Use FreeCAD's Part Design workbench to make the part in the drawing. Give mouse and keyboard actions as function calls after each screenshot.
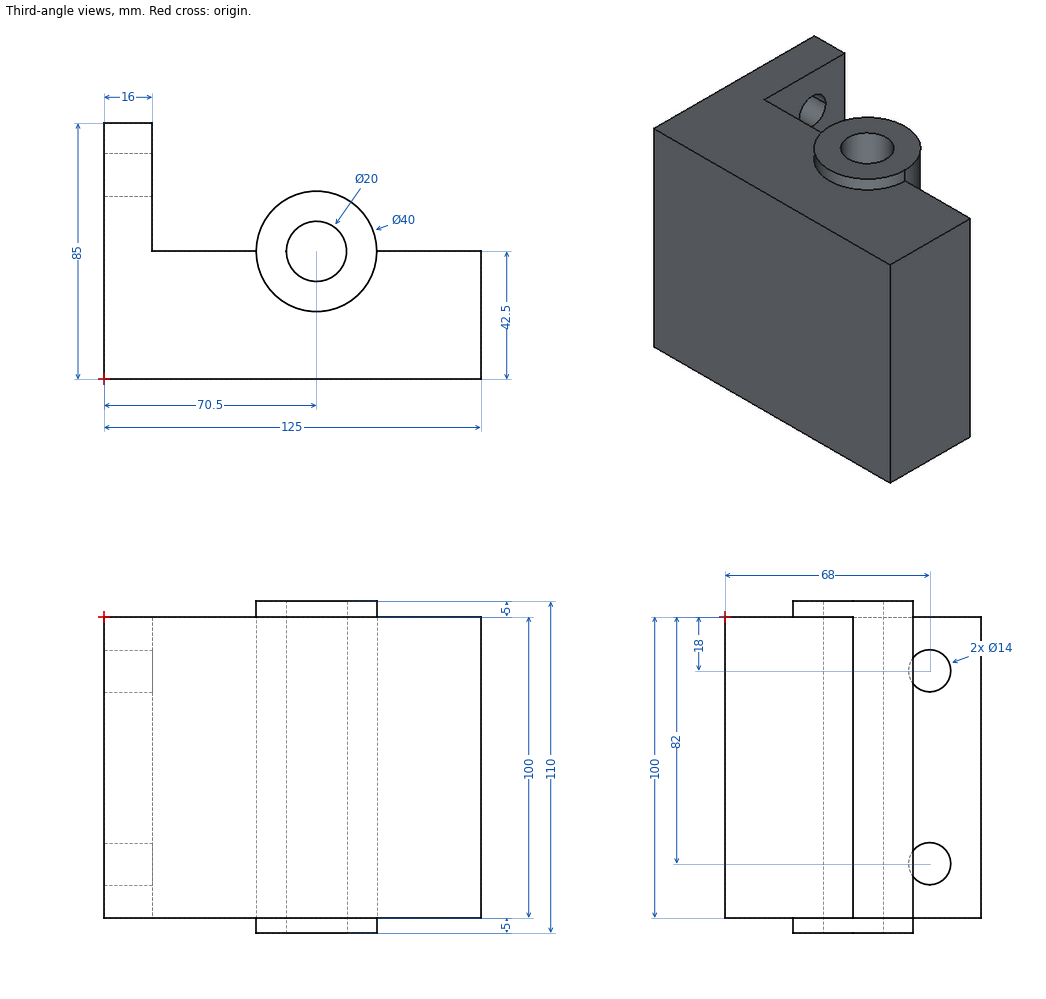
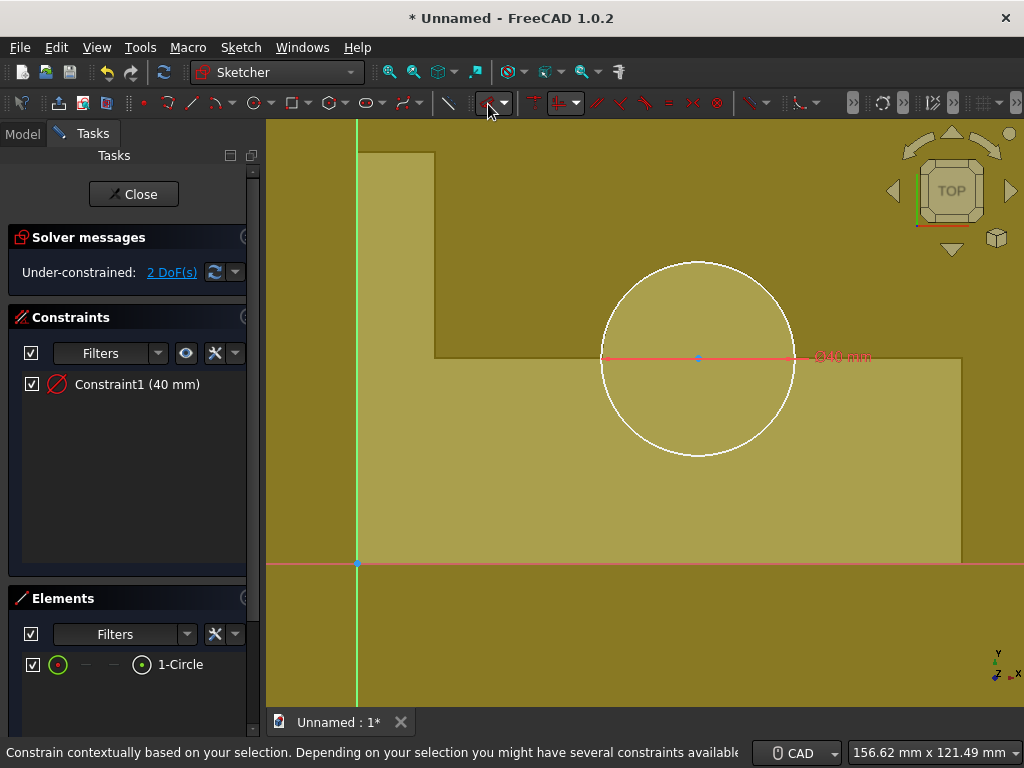
click(698, 359)
click(528, 598)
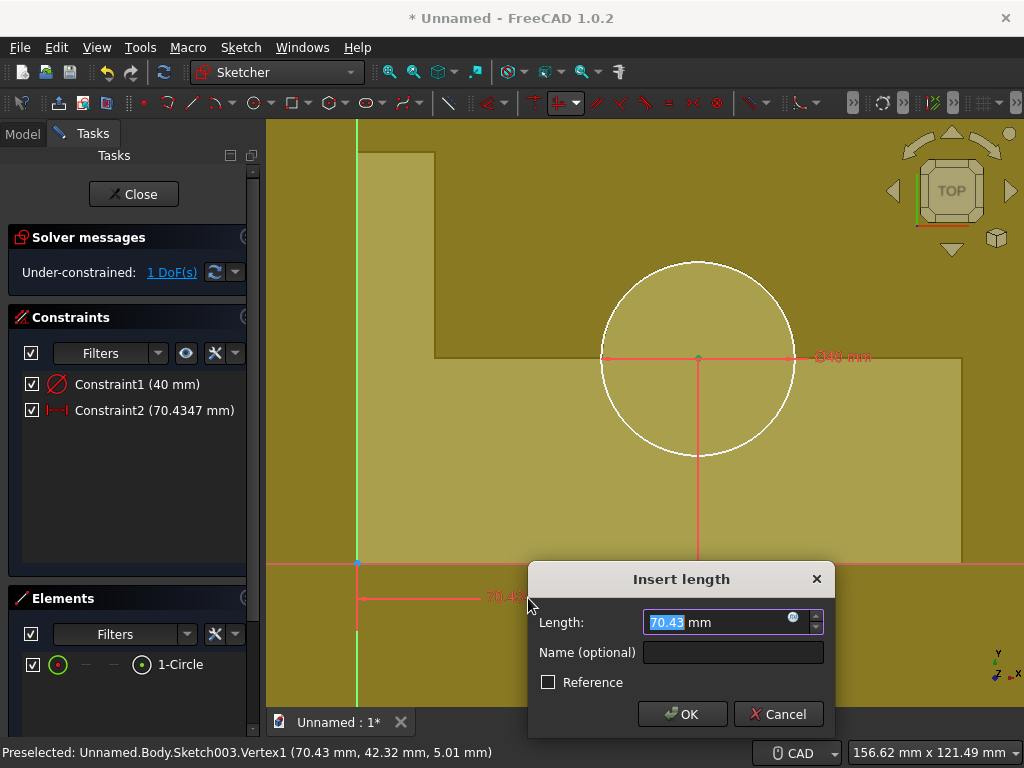
text(70.5)
key(Return)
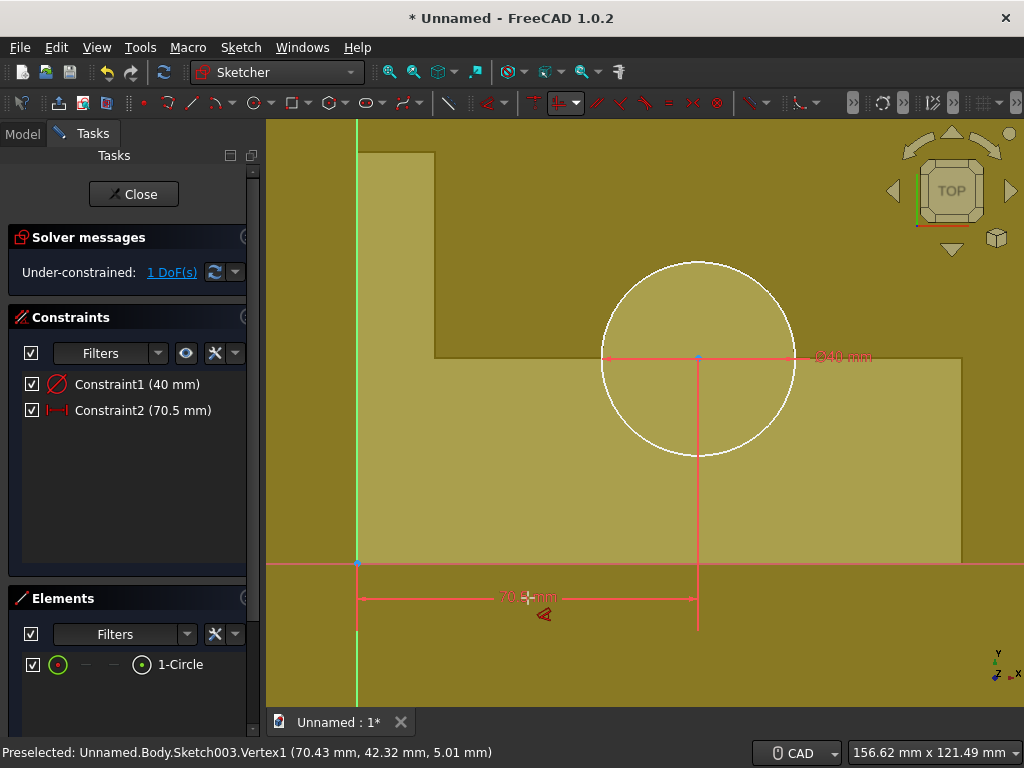
click(698, 359)
click(323, 461)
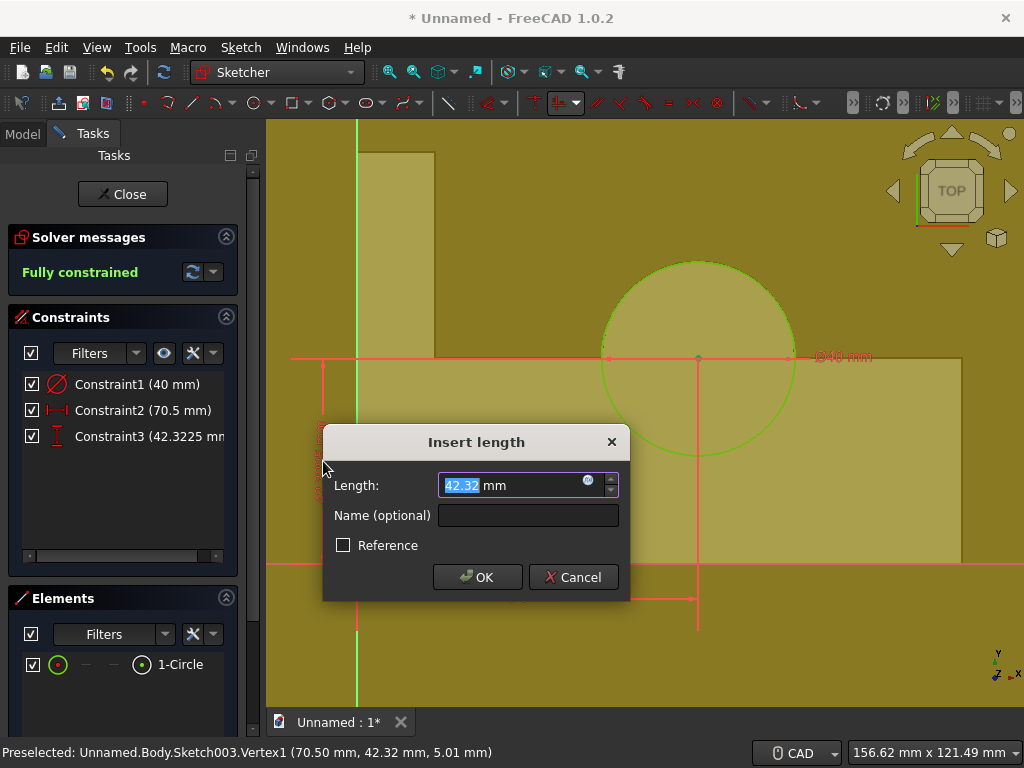
text(42.5)
key(Return)
key(Escape)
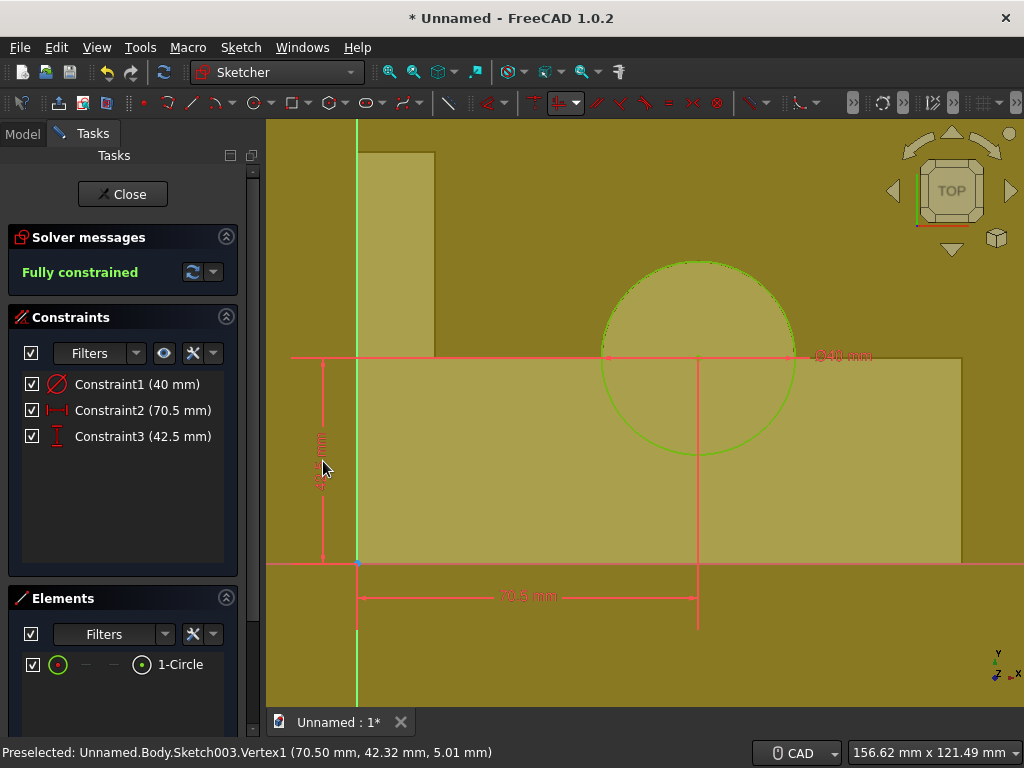
click(123, 194)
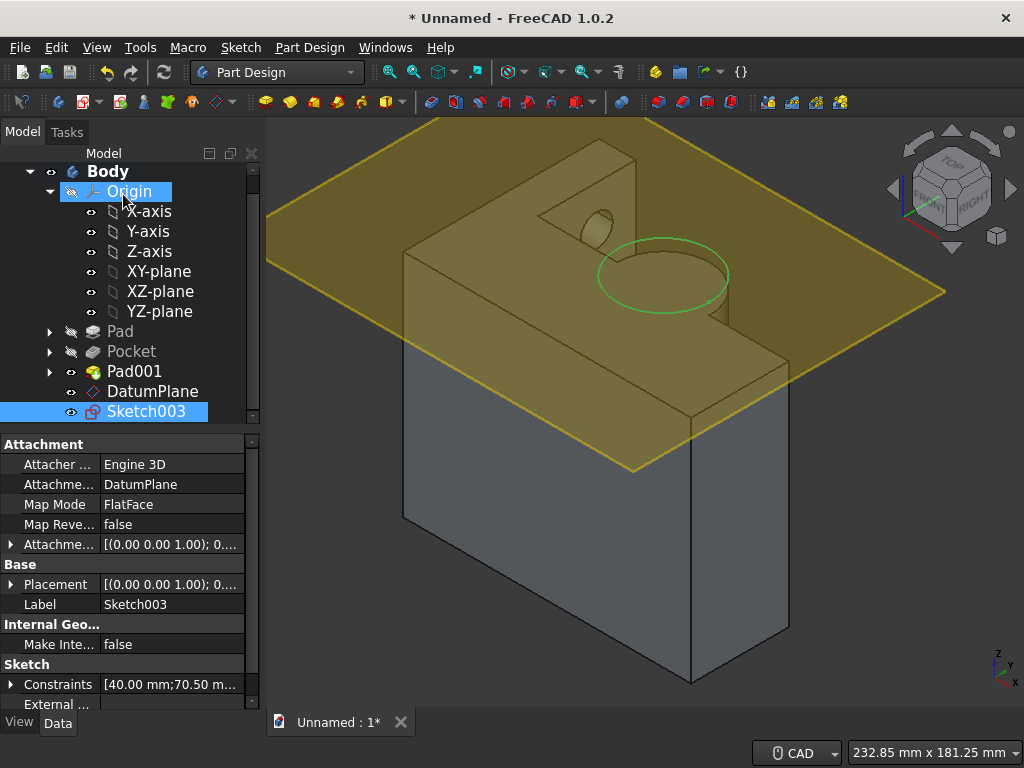
click(266, 102)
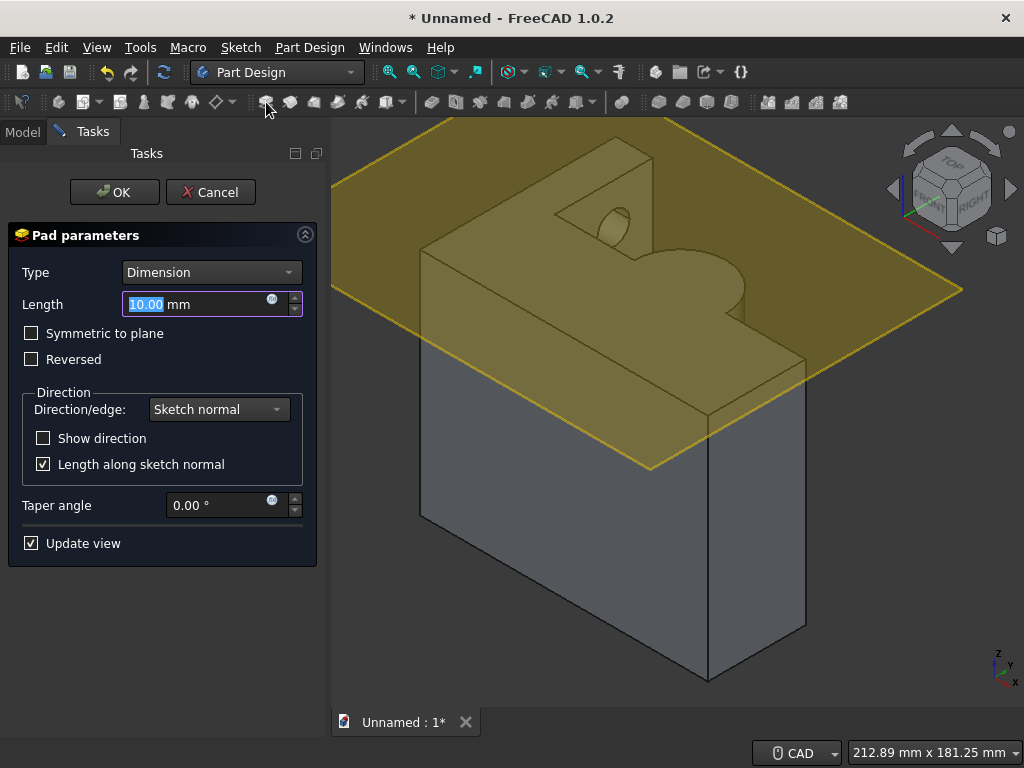
text(5)
key(Tab)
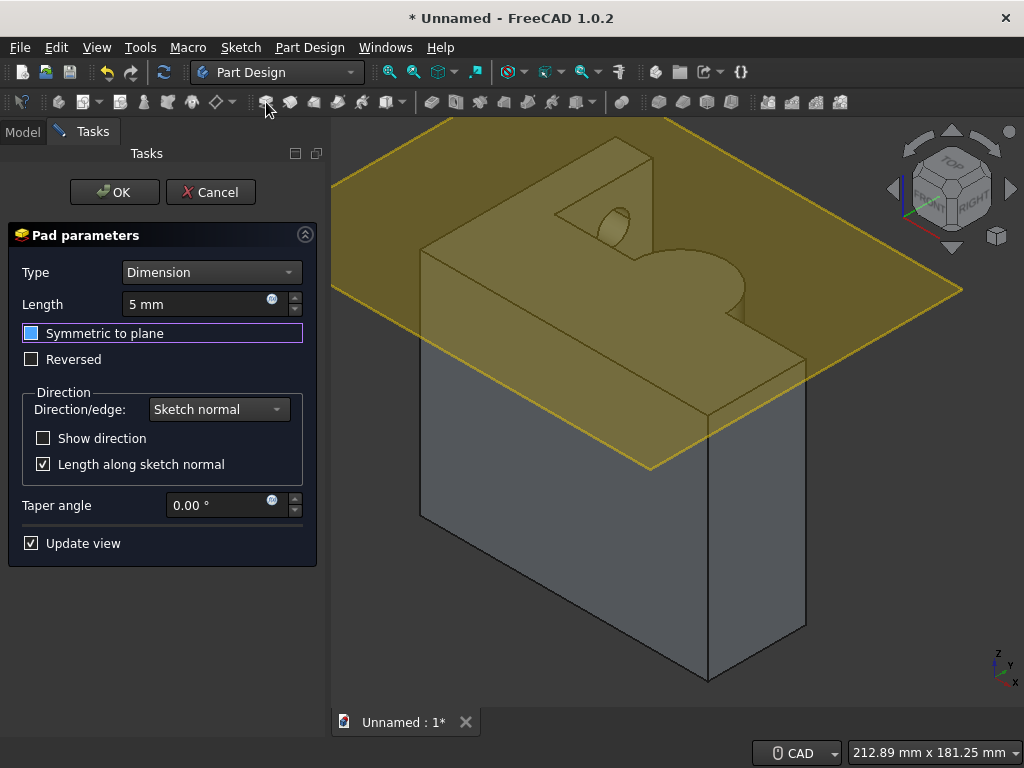
click(30, 359)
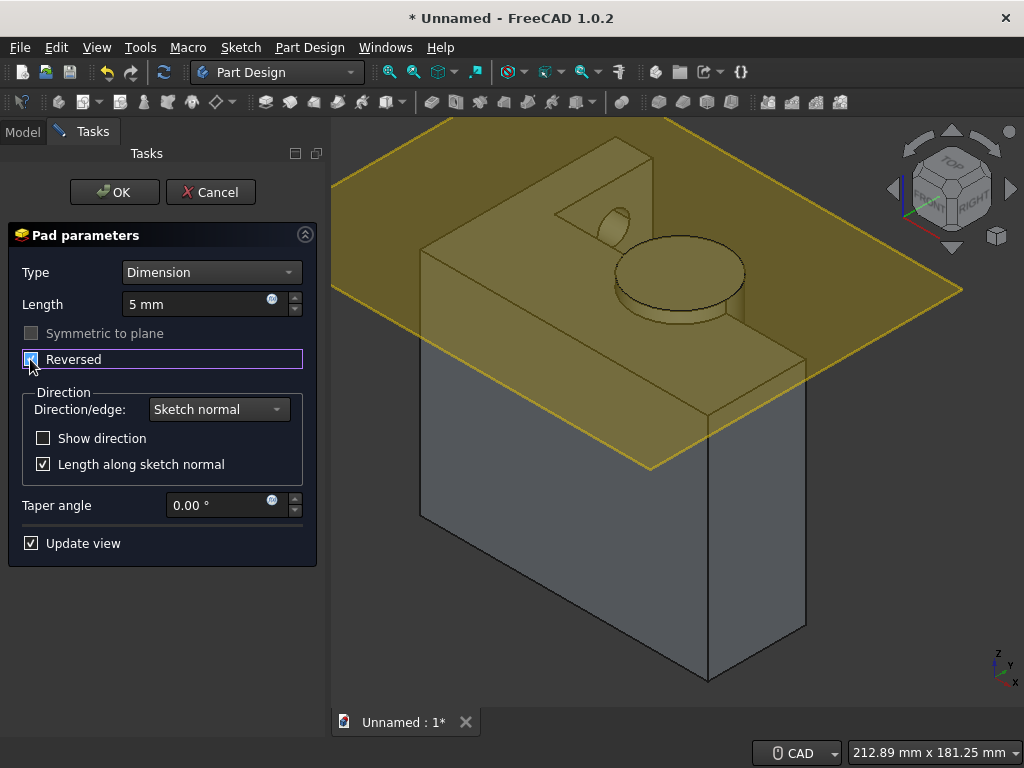
click(115, 192)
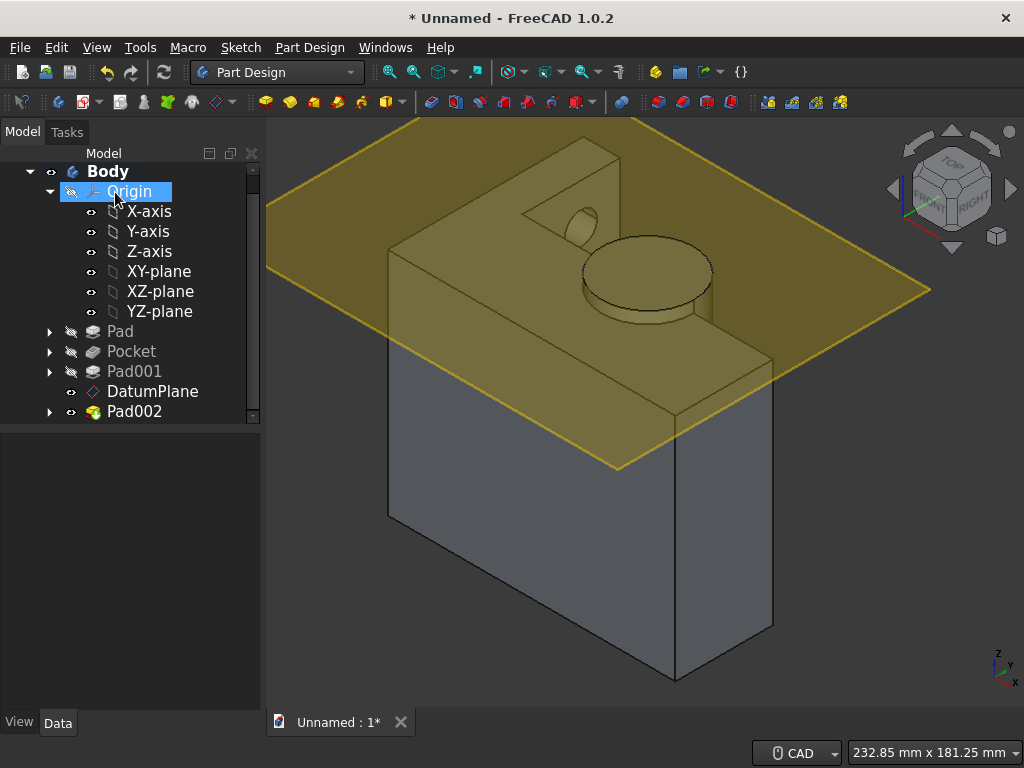
click(116, 392)
key(space)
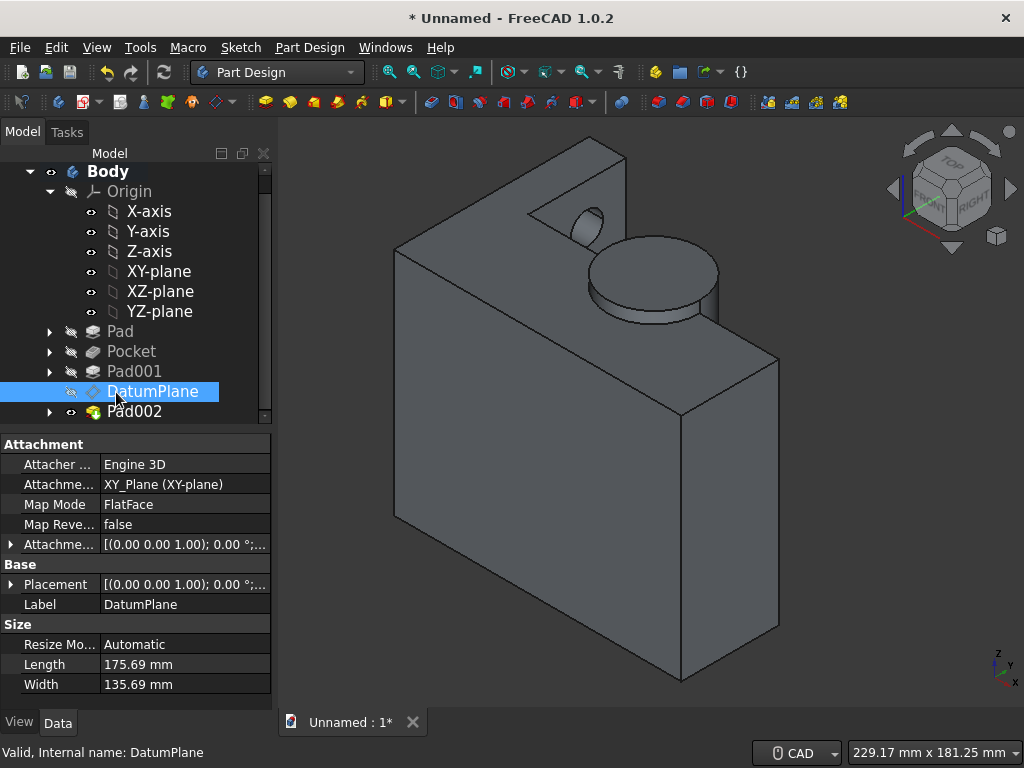
key(5)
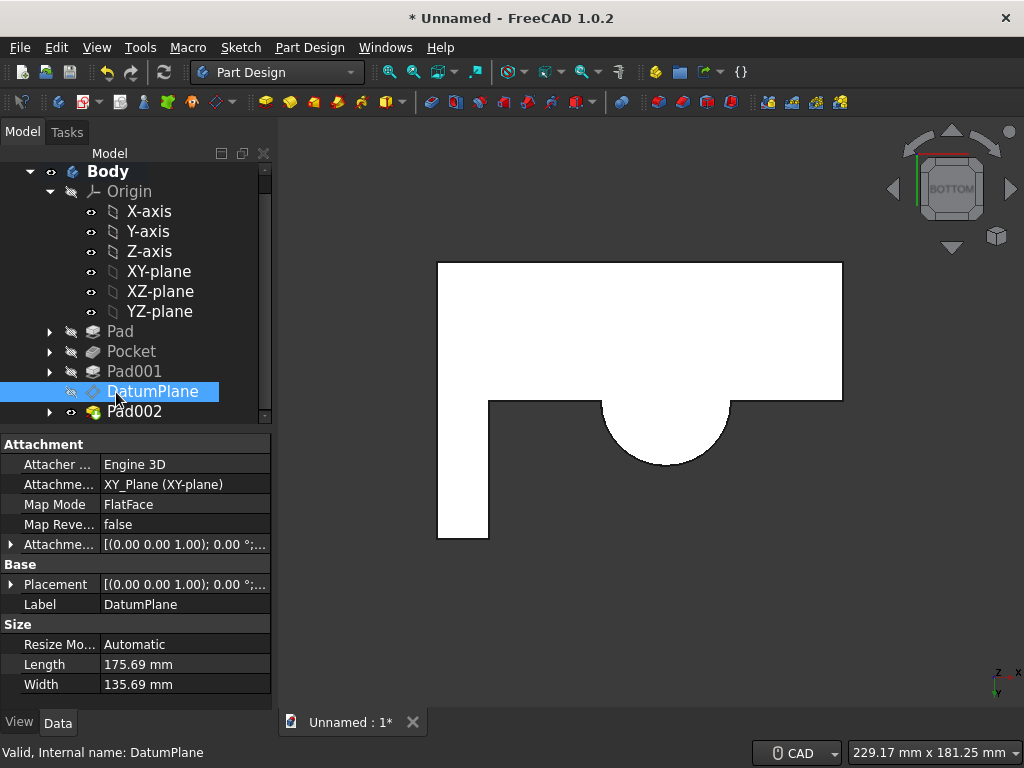
click(756, 321)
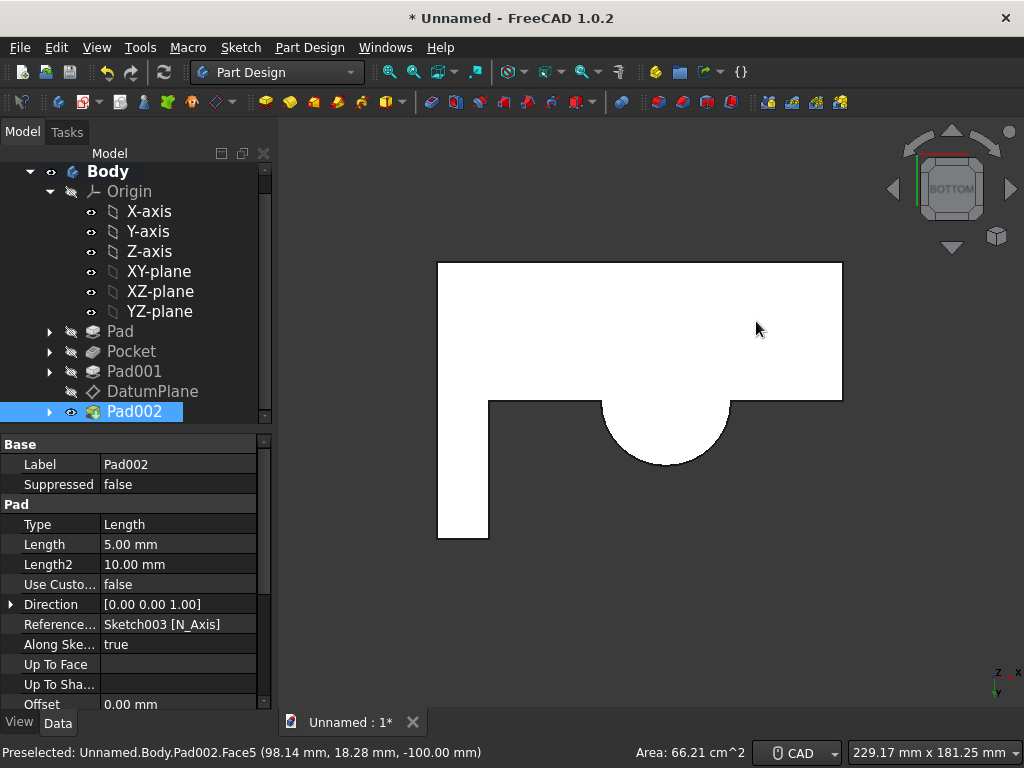
click(84, 102)